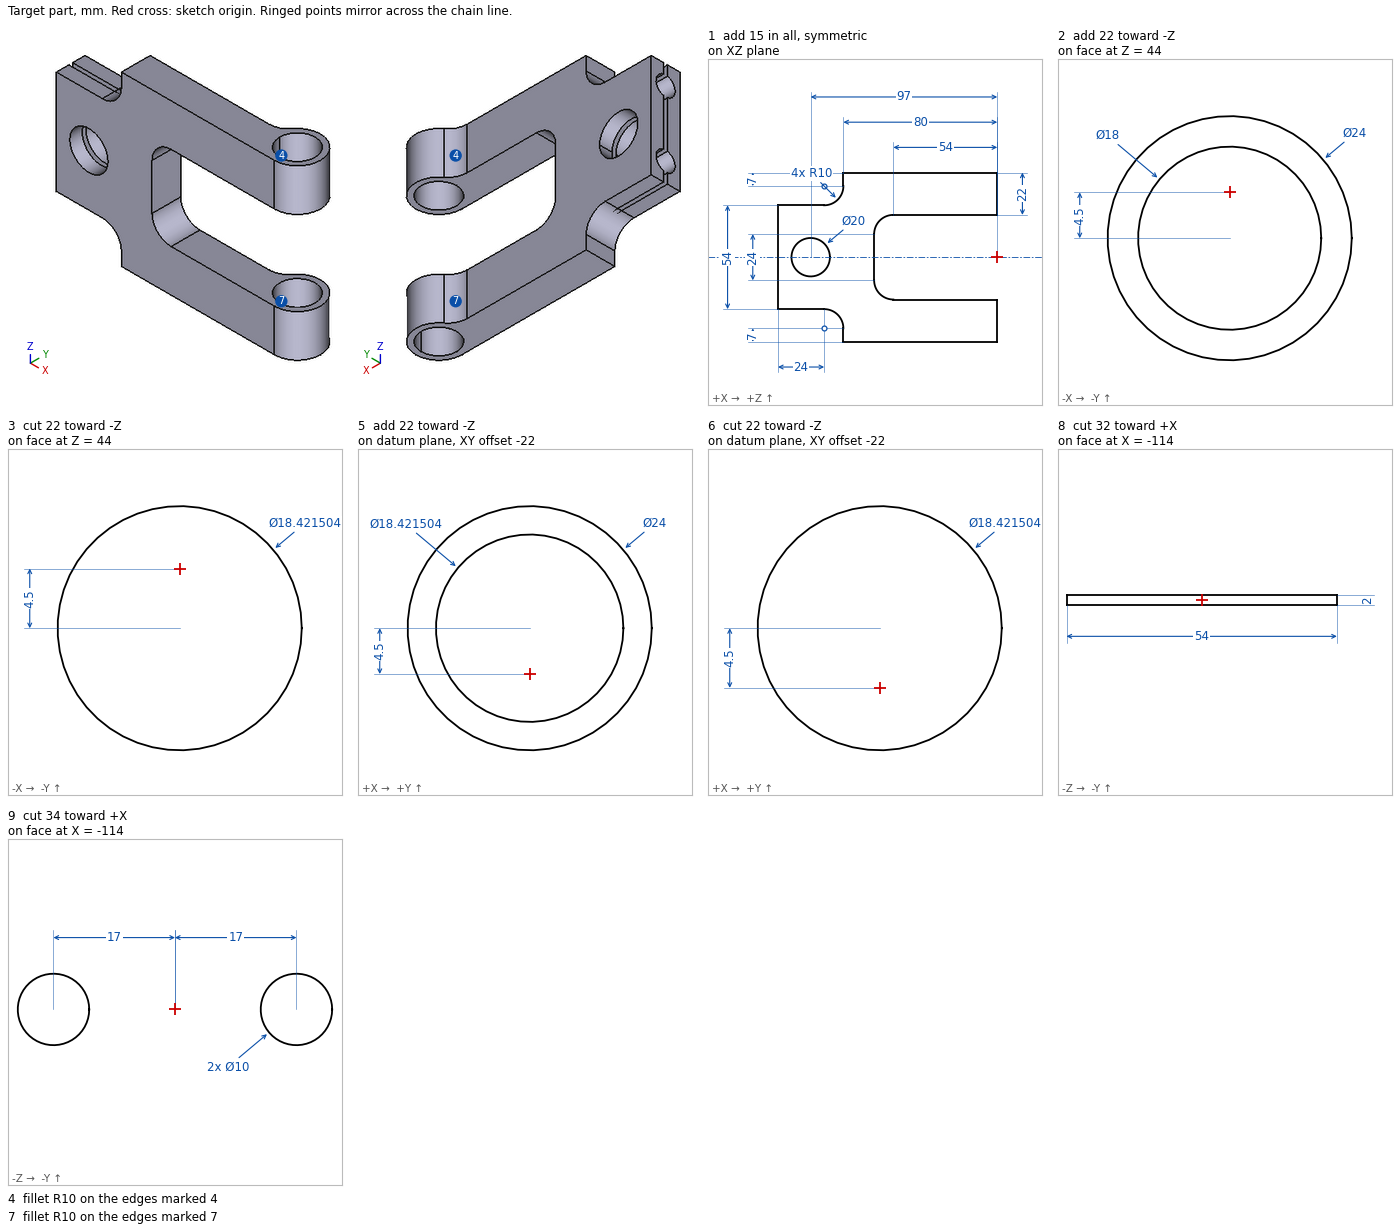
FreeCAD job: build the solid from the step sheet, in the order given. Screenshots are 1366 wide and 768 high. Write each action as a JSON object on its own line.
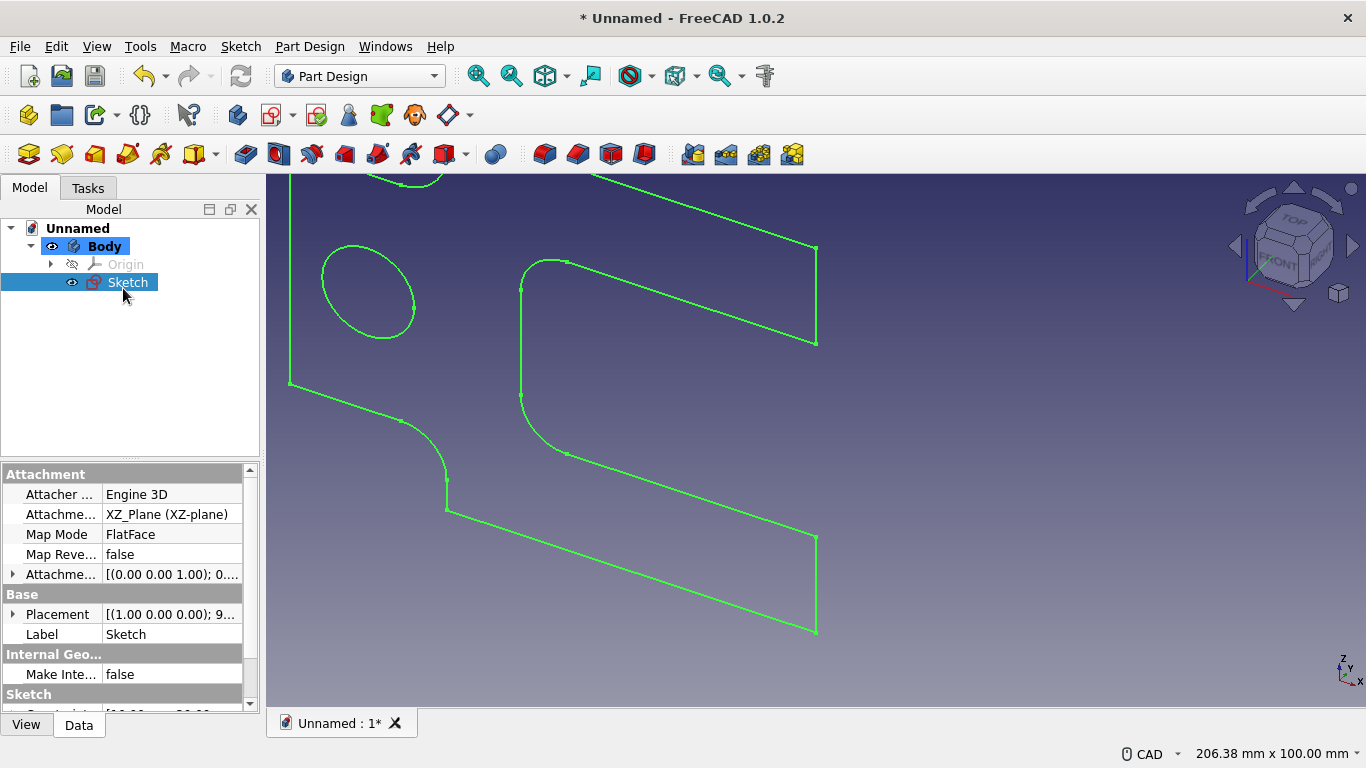
{"action": "left_click", "coordinate": [29, 154]}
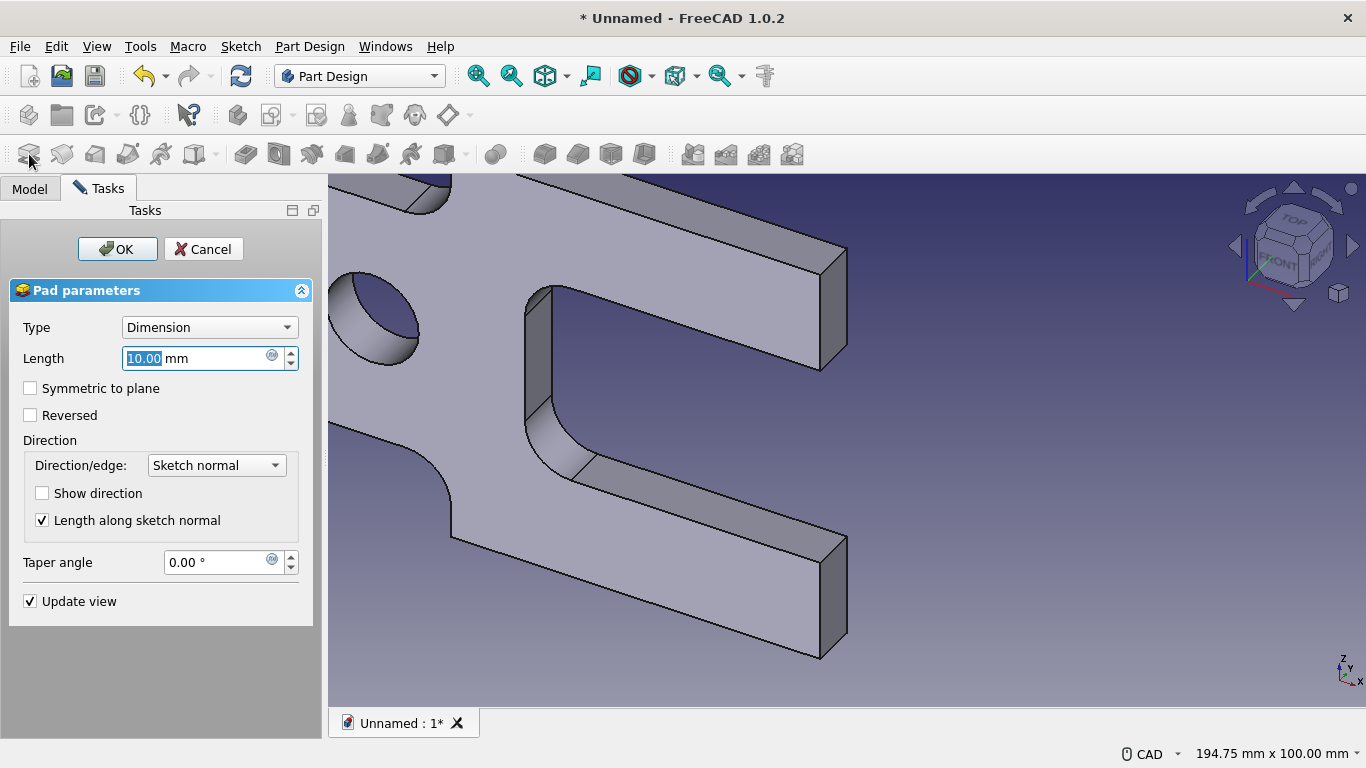
{"action": "type", "text": "15"}
{"action": "key", "text": "Tab"}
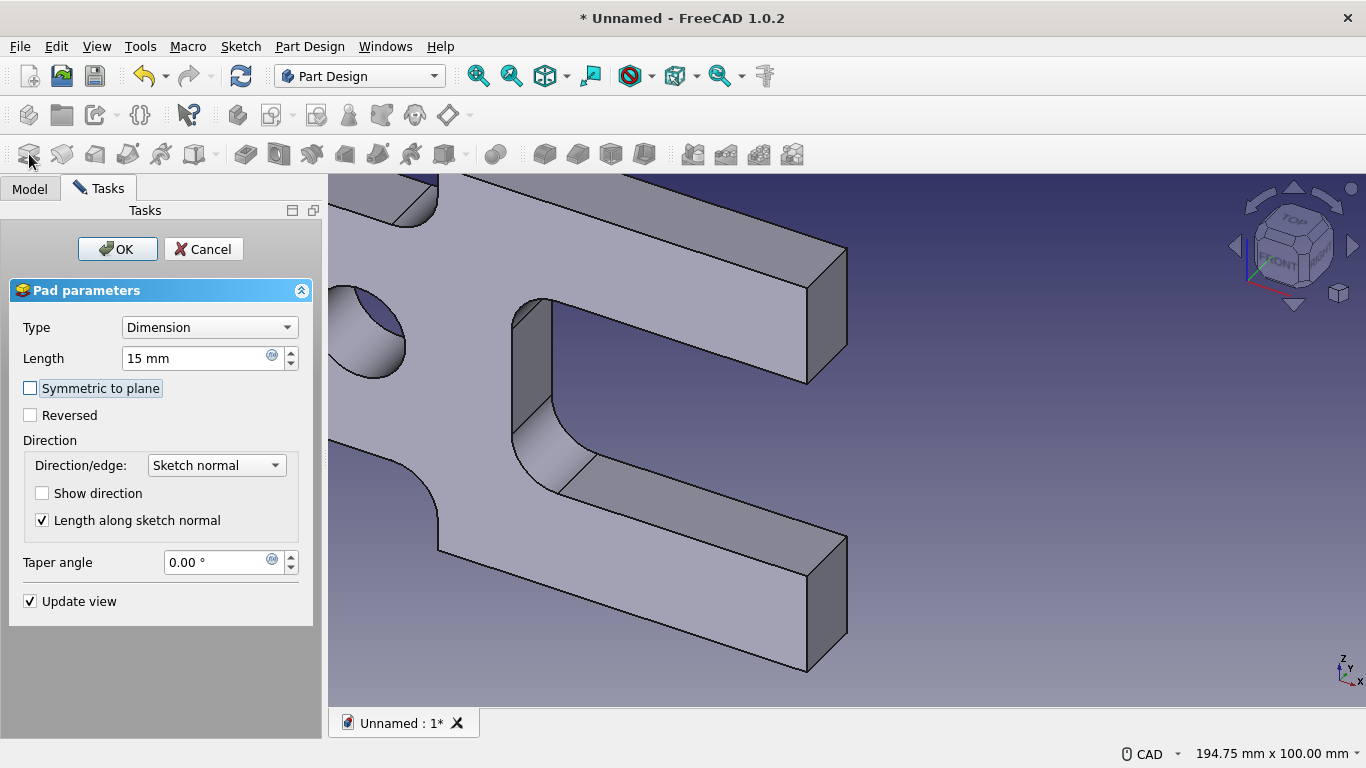
{"action": "left_click", "coordinate": [31, 388]}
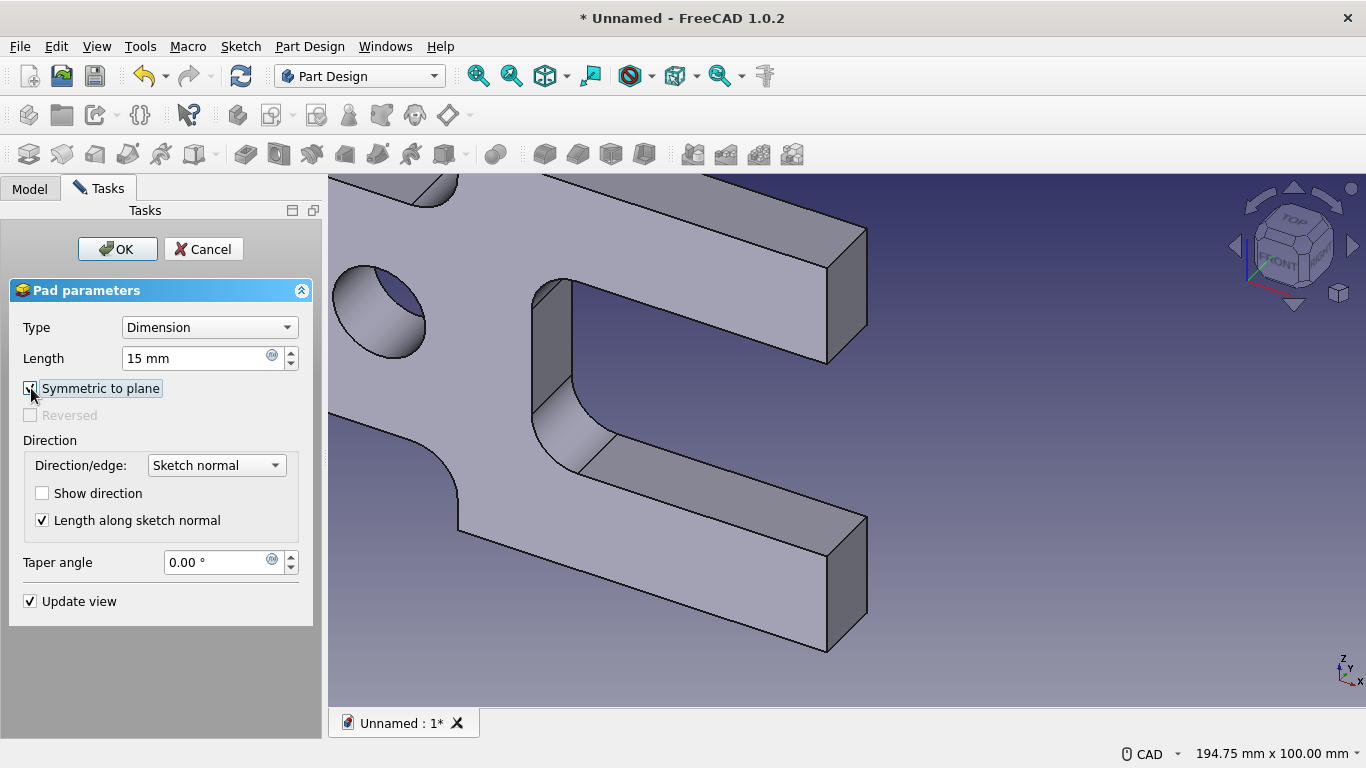
{"action": "left_click", "coordinate": [118, 249]}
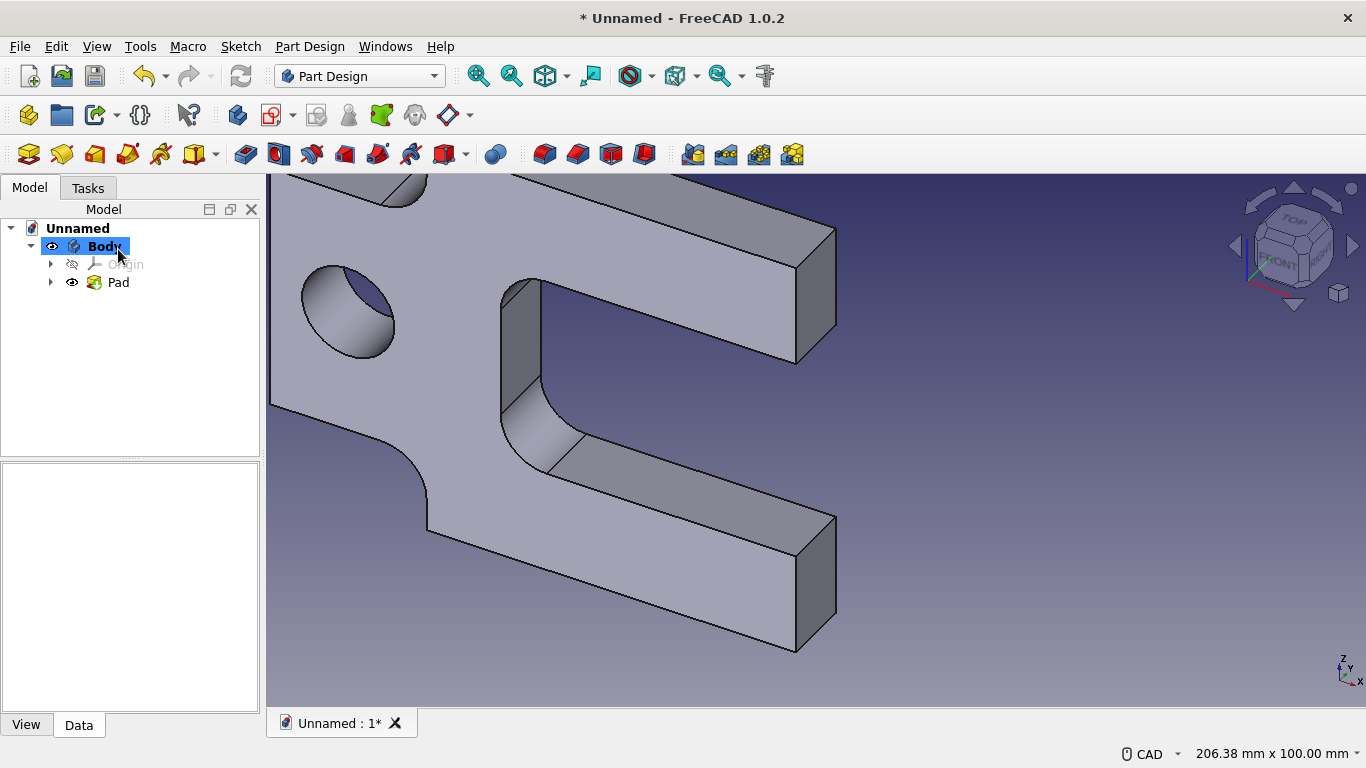
{"action": "left_click", "coordinate": [479, 76]}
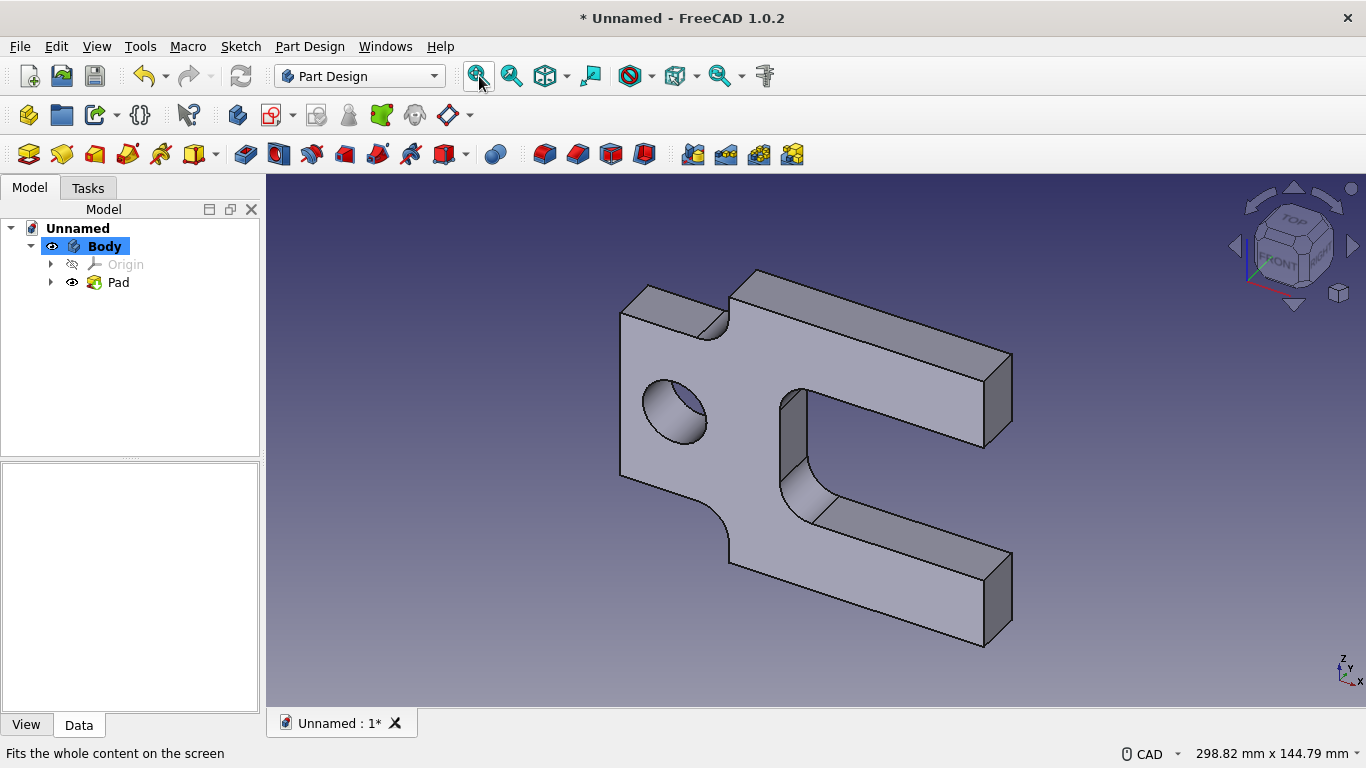
{"action": "left_click", "coordinate": [943, 349]}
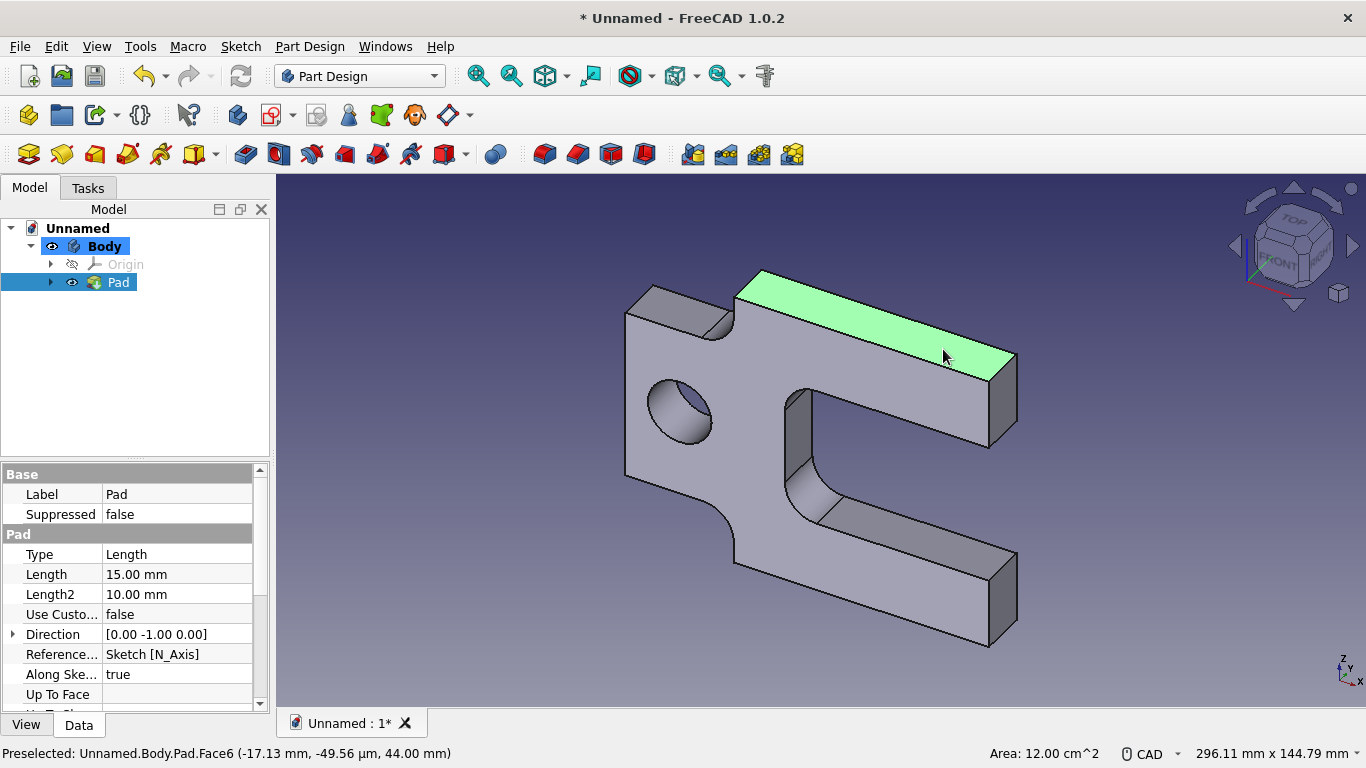
{"action": "left_click", "coordinate": [270, 116]}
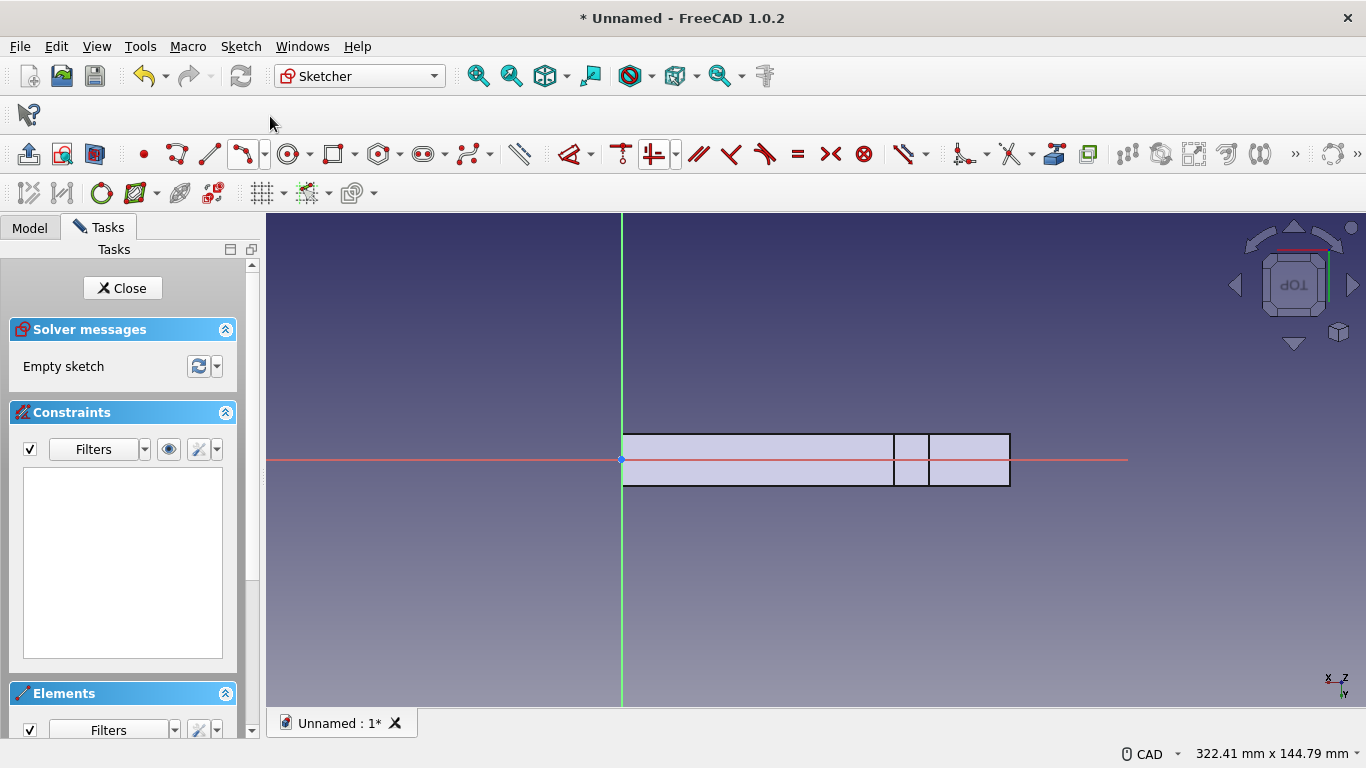
{"action": "scroll", "coordinate": [580, 480], "scroll_direction": "up", "scroll_amount": 7}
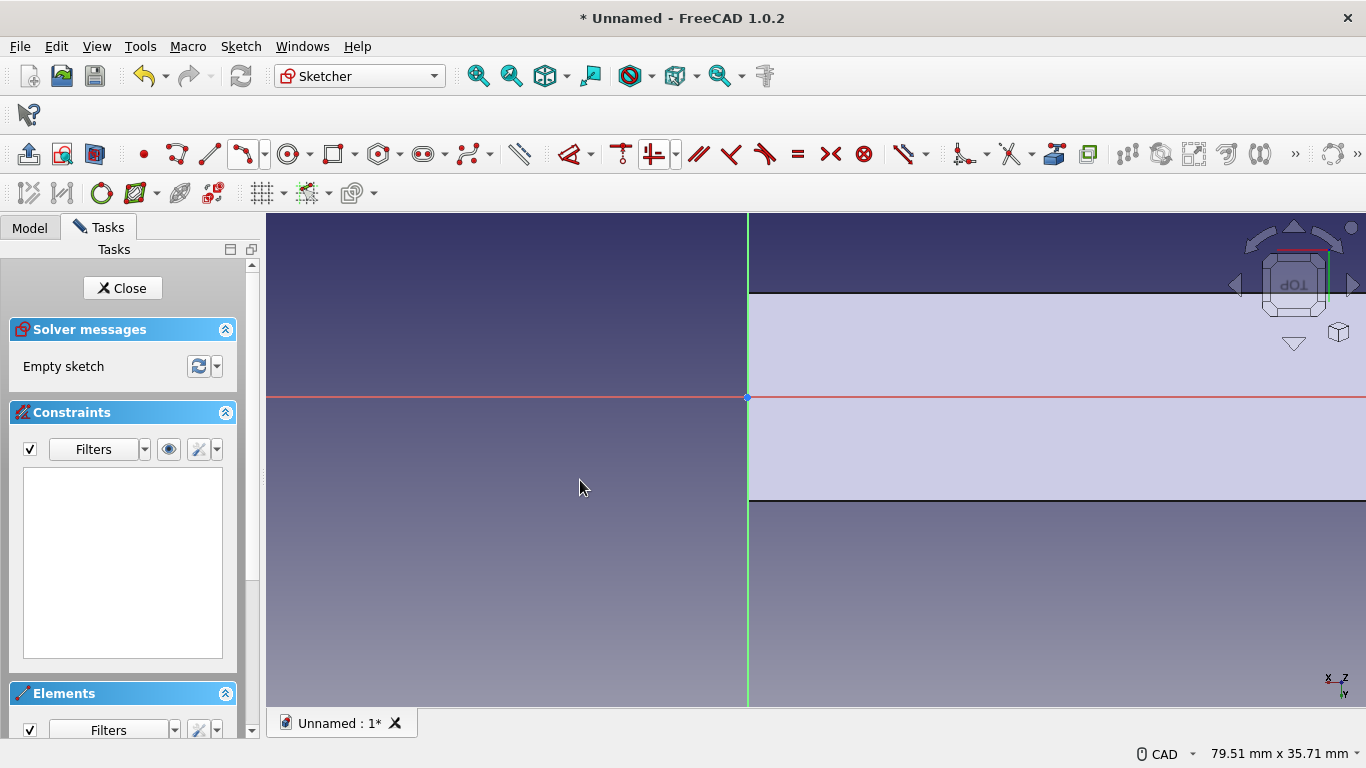
{"action": "left_click", "coordinate": [288, 154]}